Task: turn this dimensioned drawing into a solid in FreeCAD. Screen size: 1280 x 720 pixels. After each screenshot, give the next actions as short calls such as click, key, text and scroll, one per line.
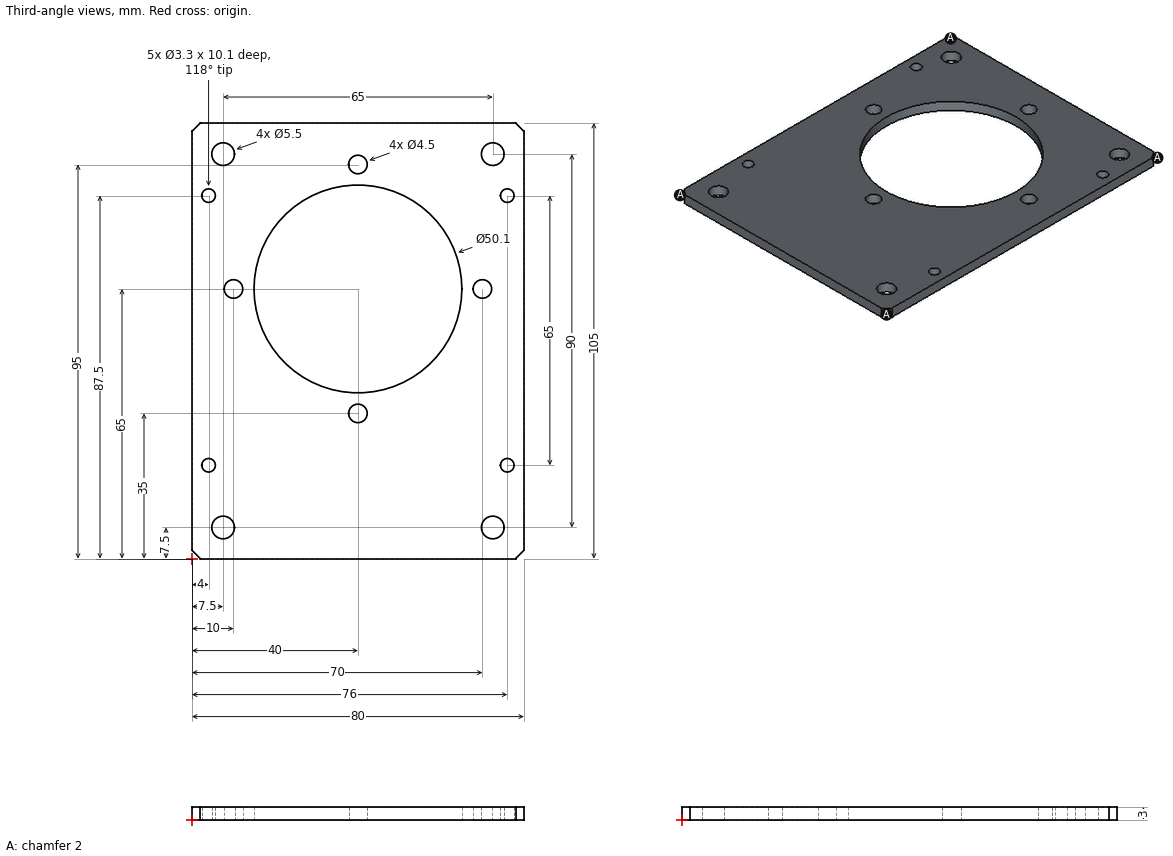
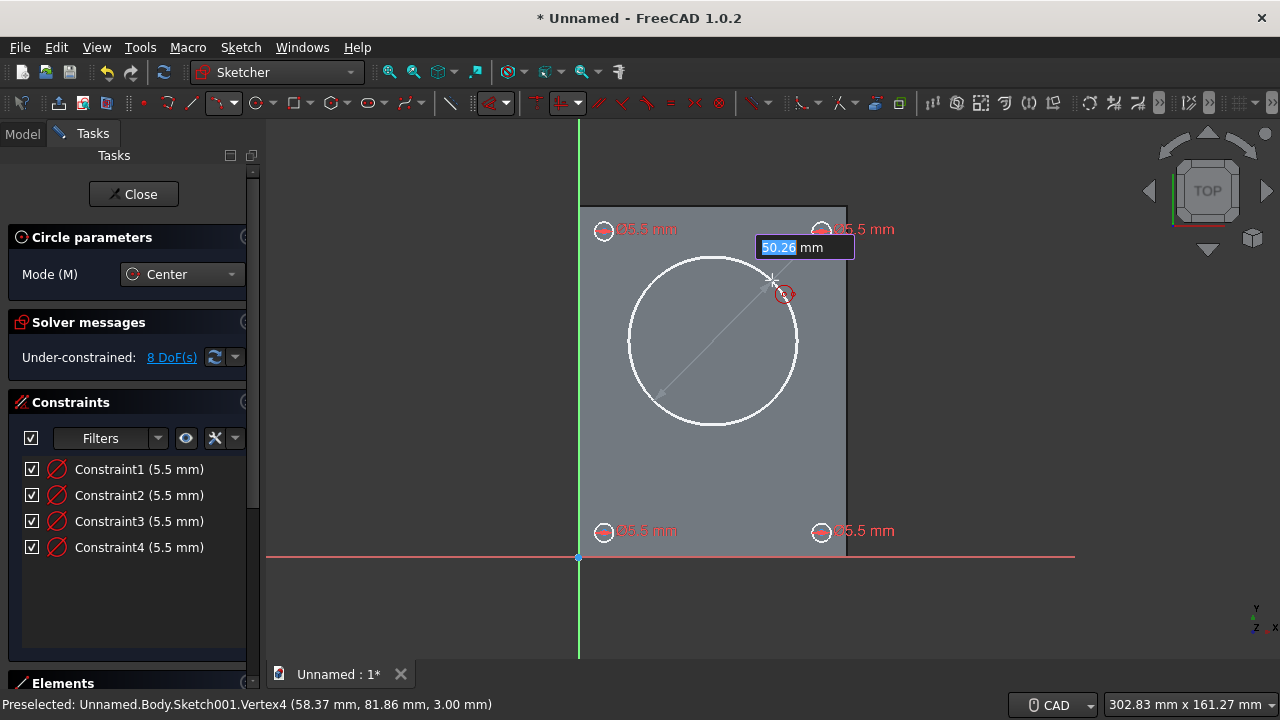
text(50.1)
key(Return)
key(Escape)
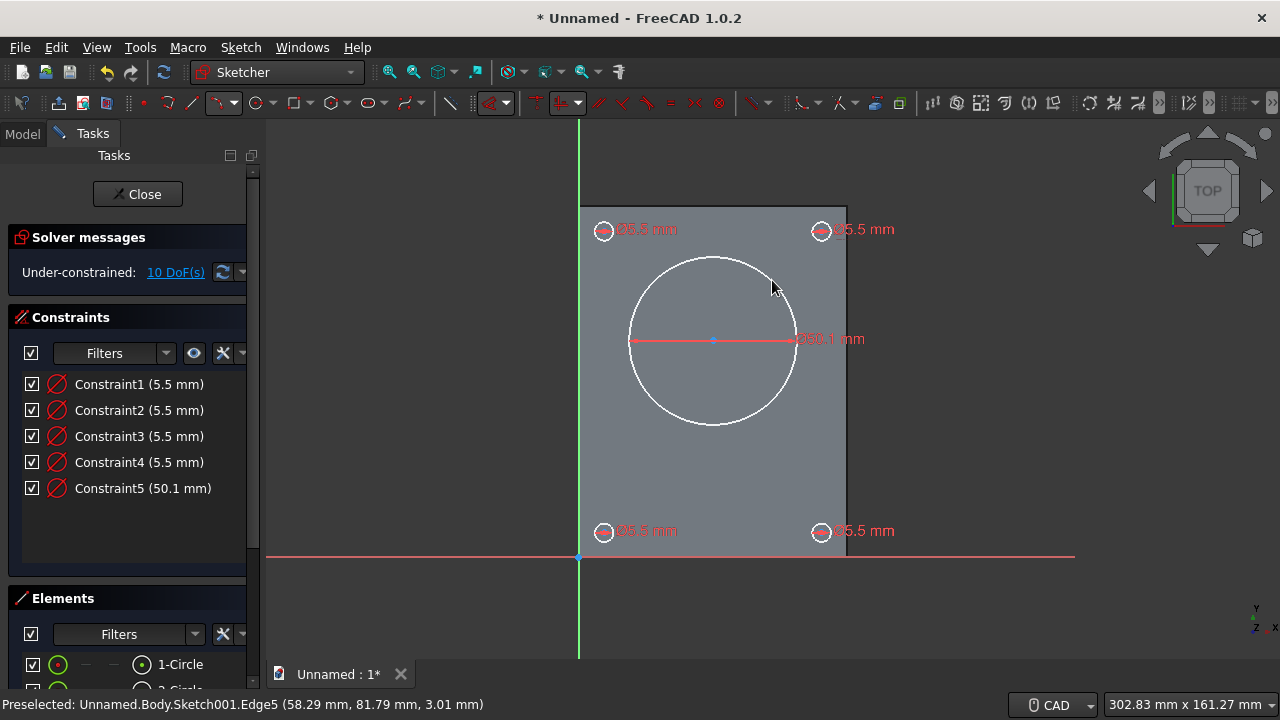
click(604, 231)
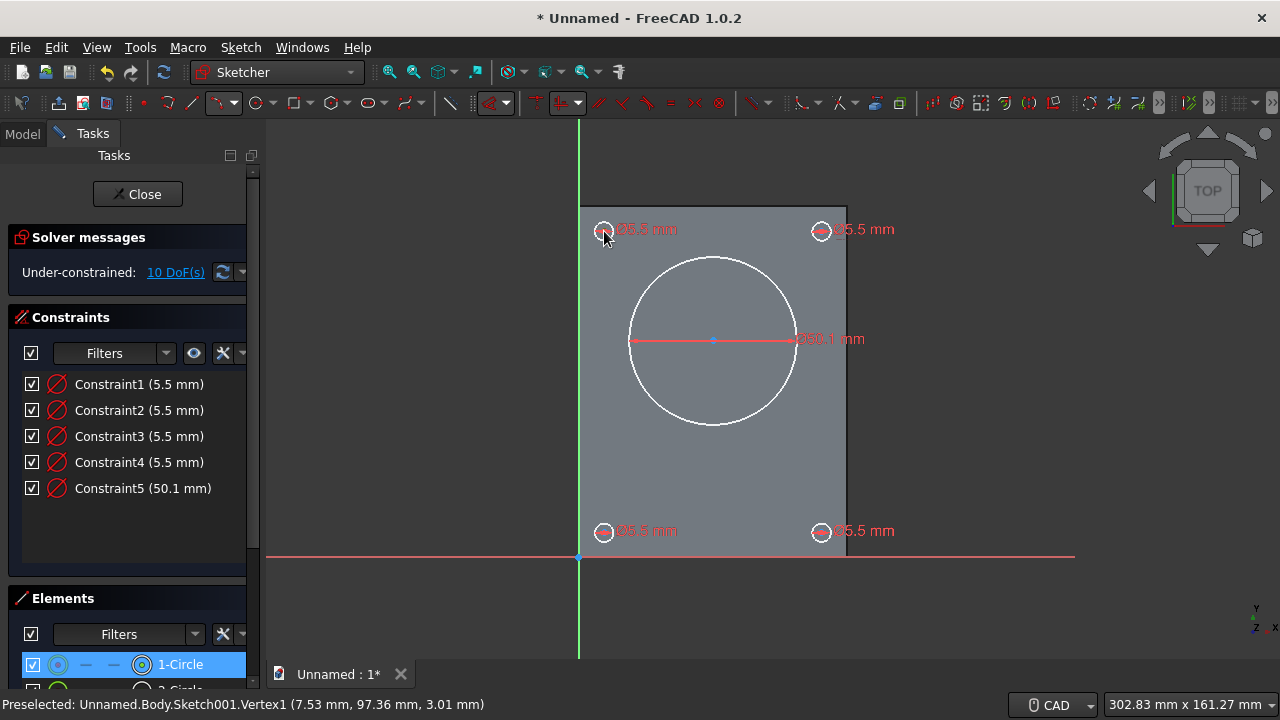
click(822, 231)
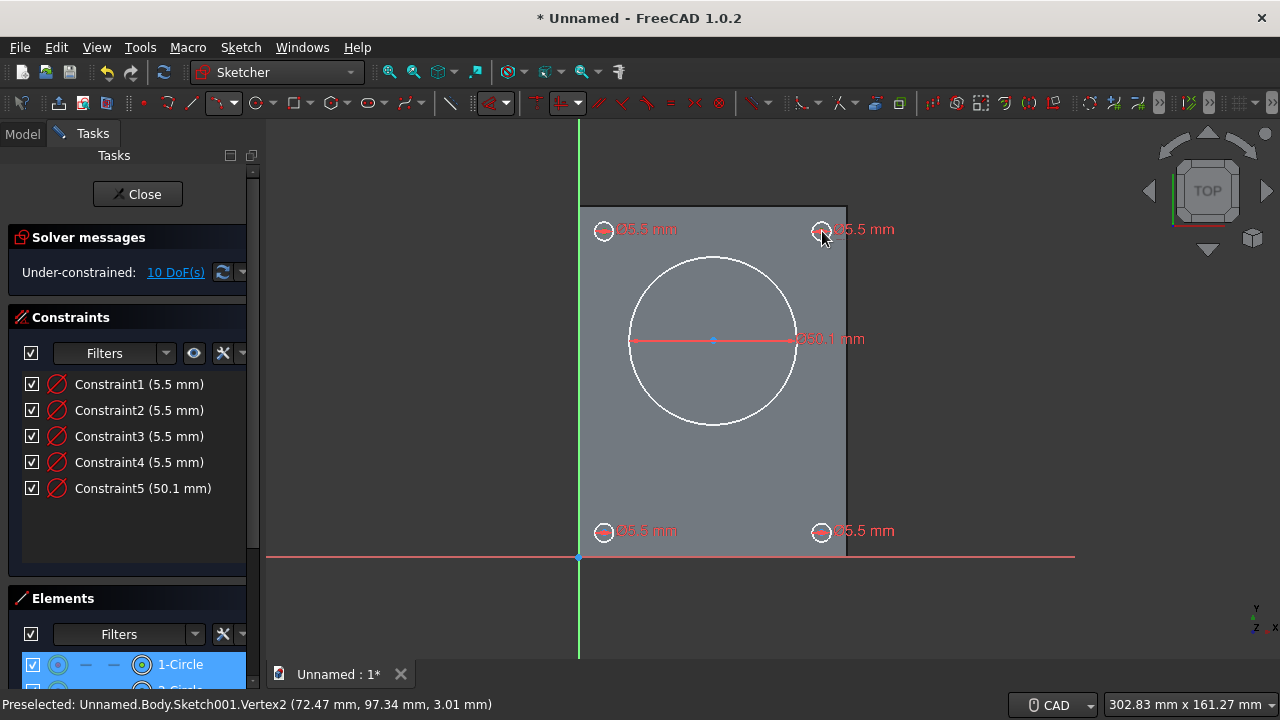
click(580, 104)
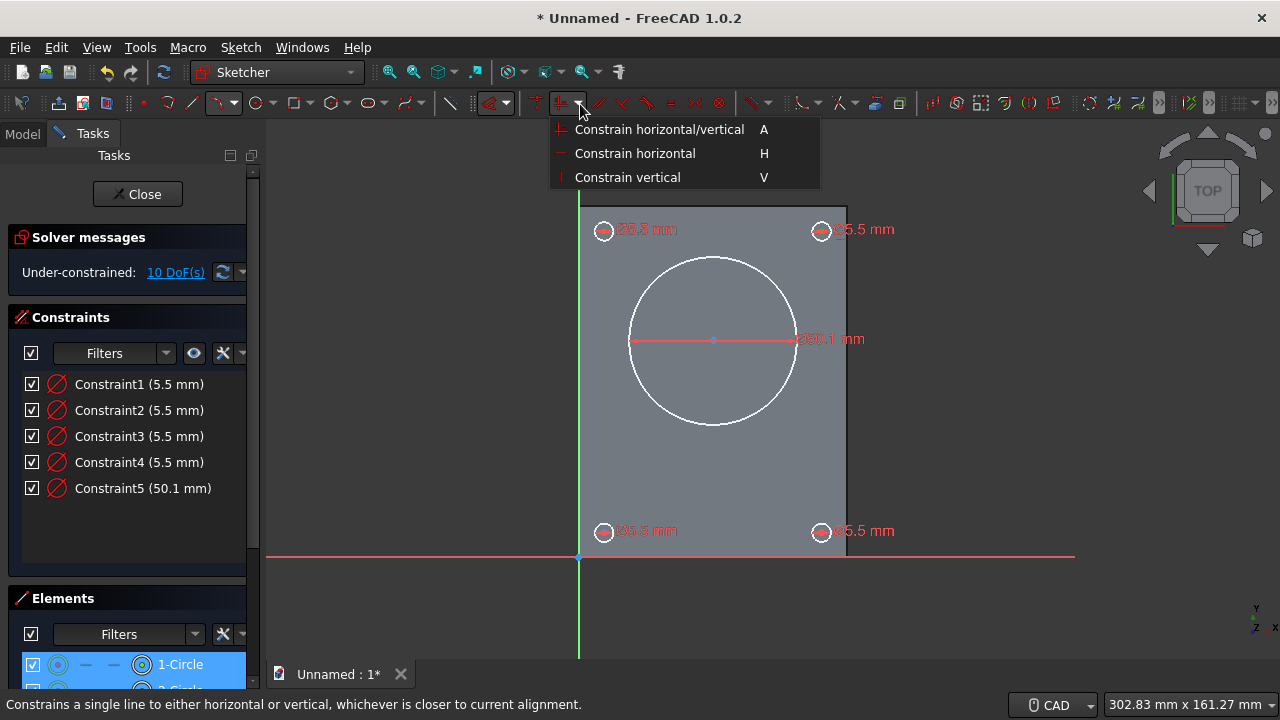
click(685, 153)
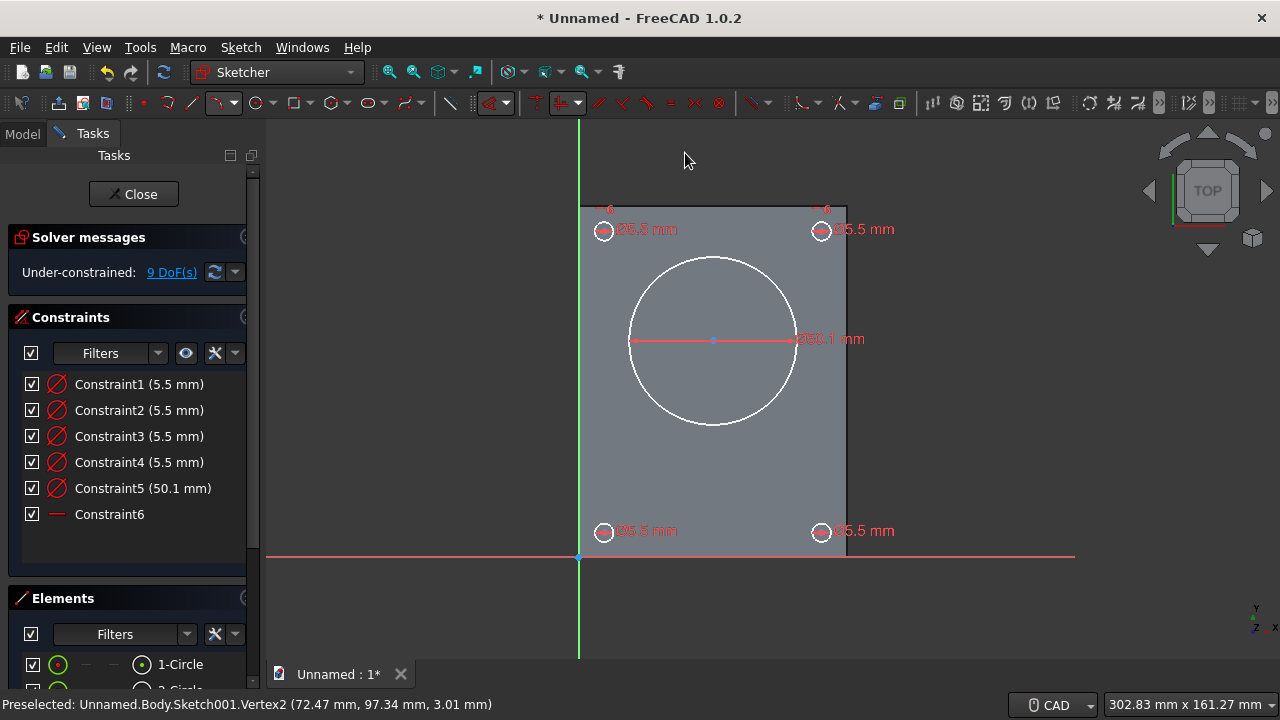
click(822, 231)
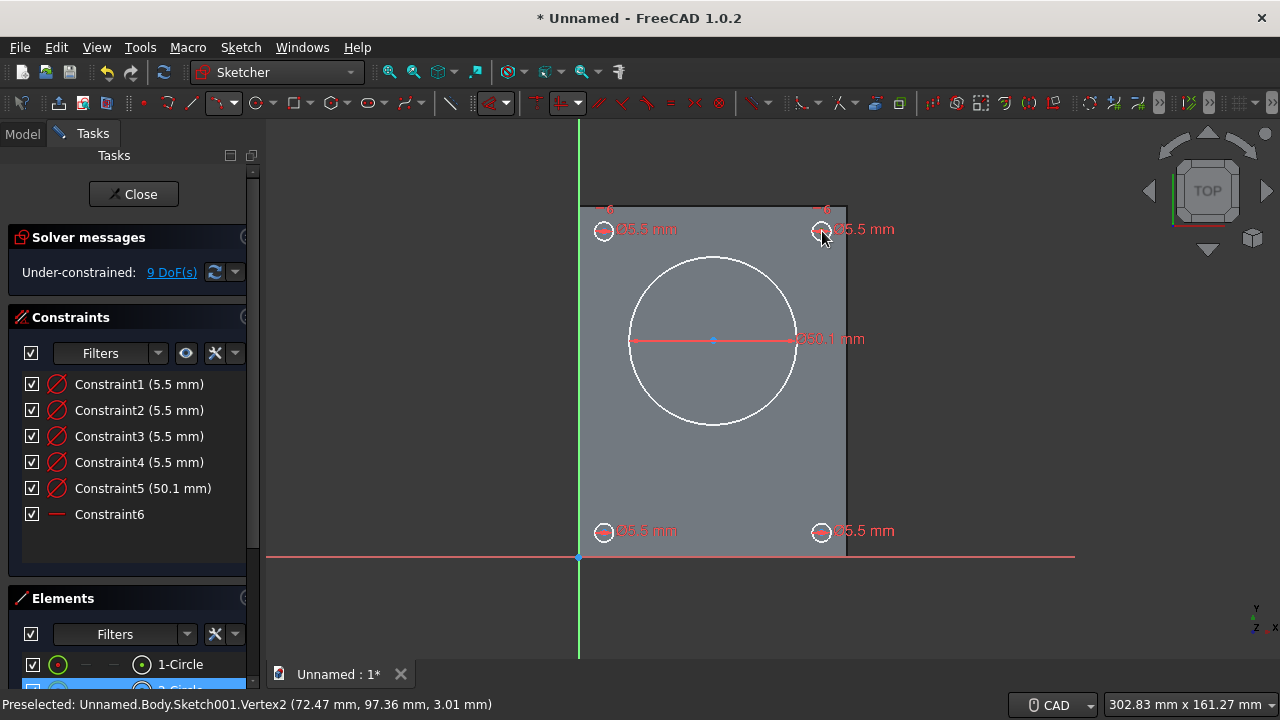
click(822, 533)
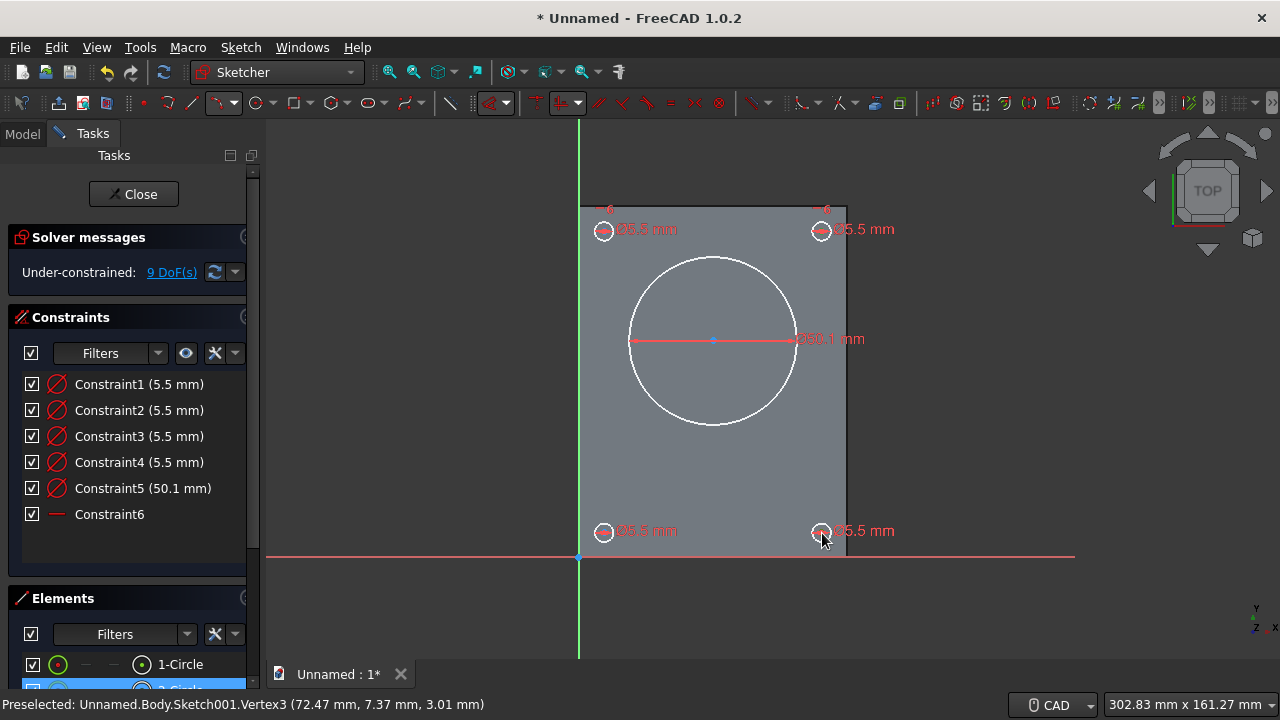
key(v)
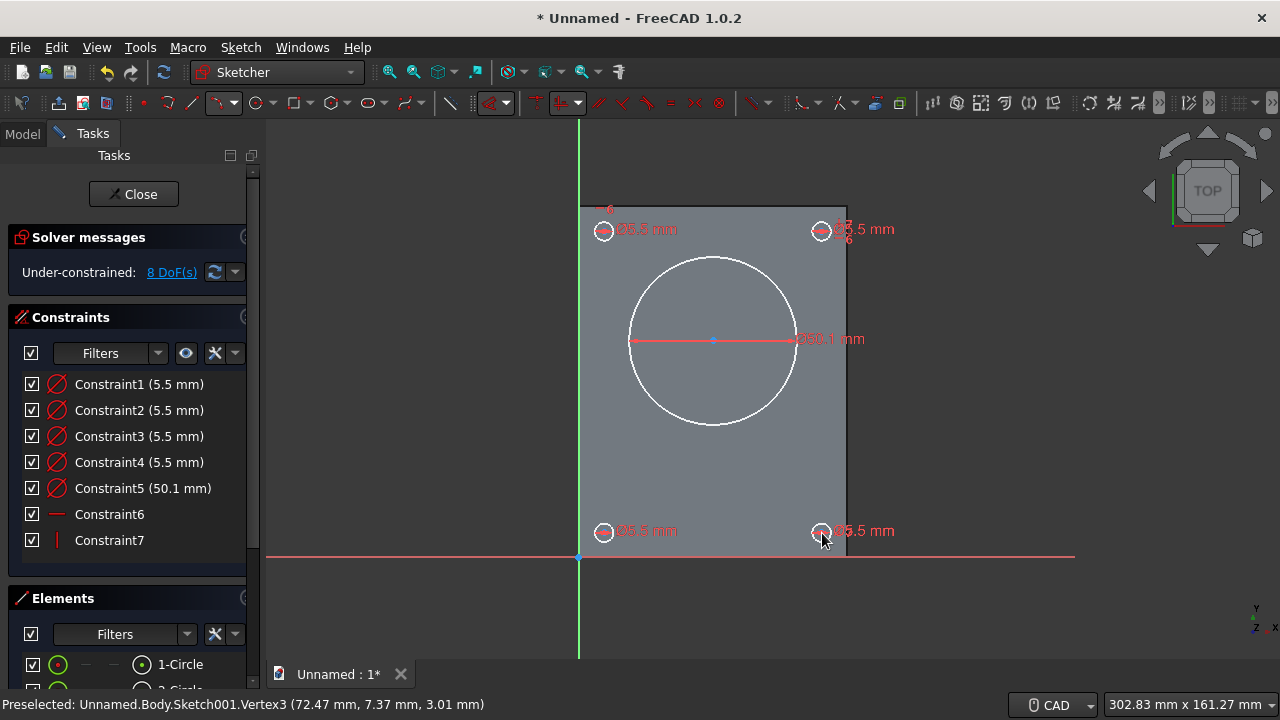
click(604, 231)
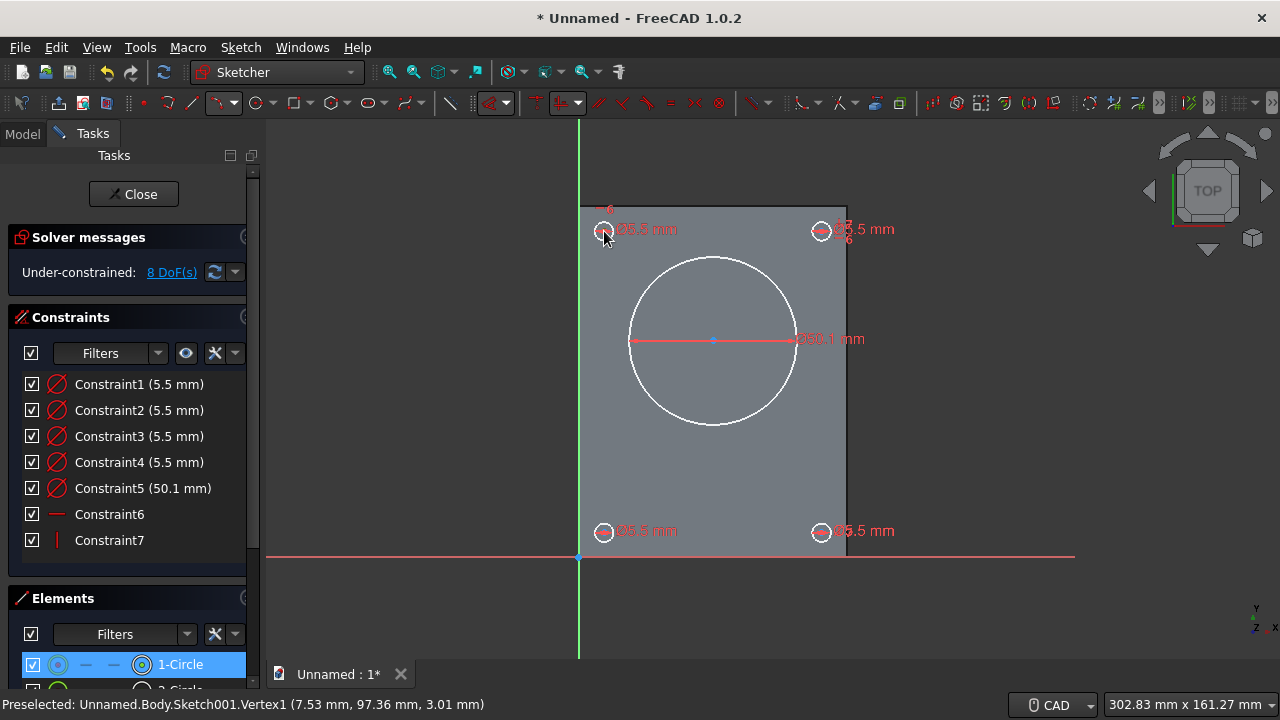
click(604, 533)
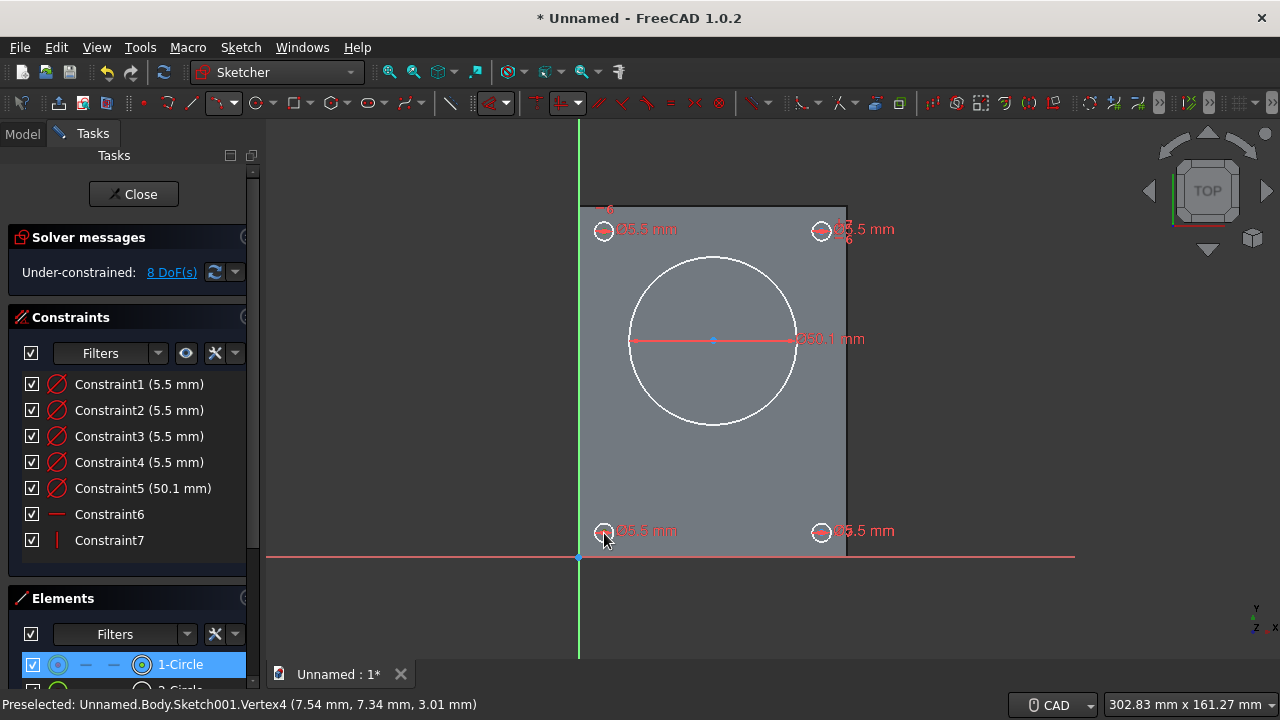
key(v)